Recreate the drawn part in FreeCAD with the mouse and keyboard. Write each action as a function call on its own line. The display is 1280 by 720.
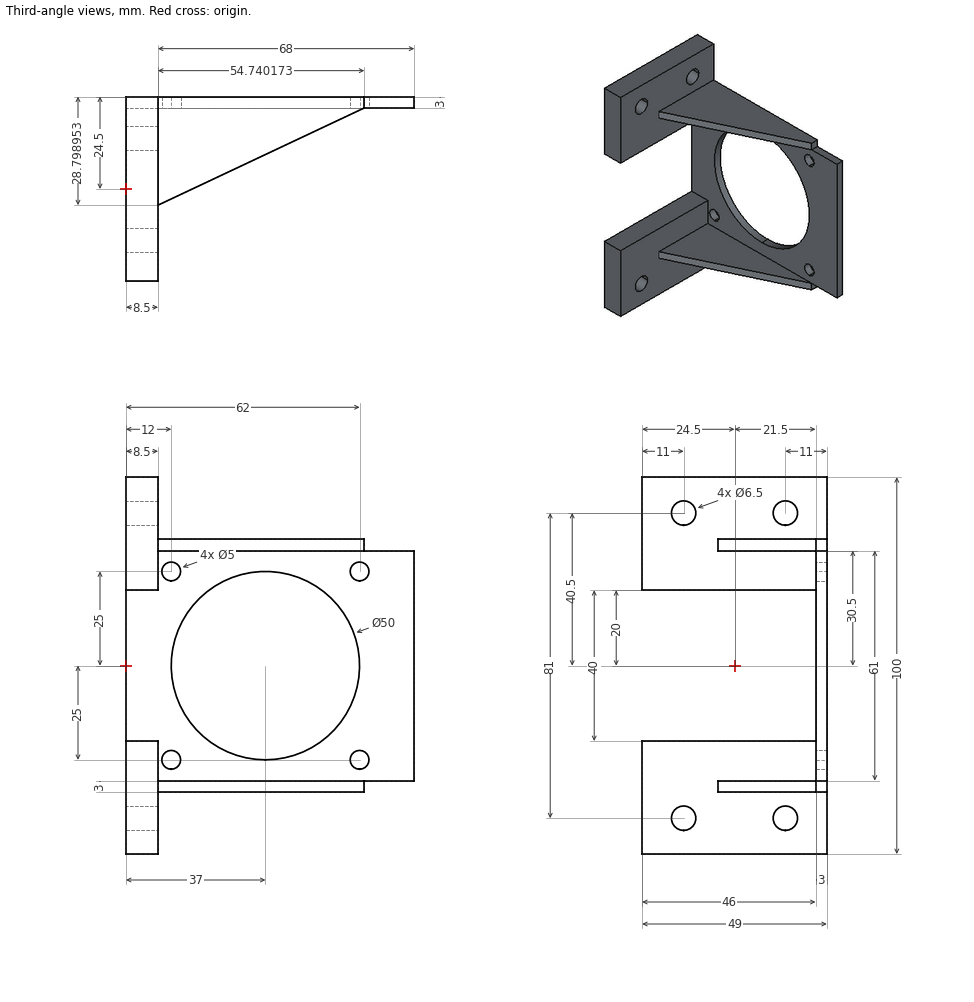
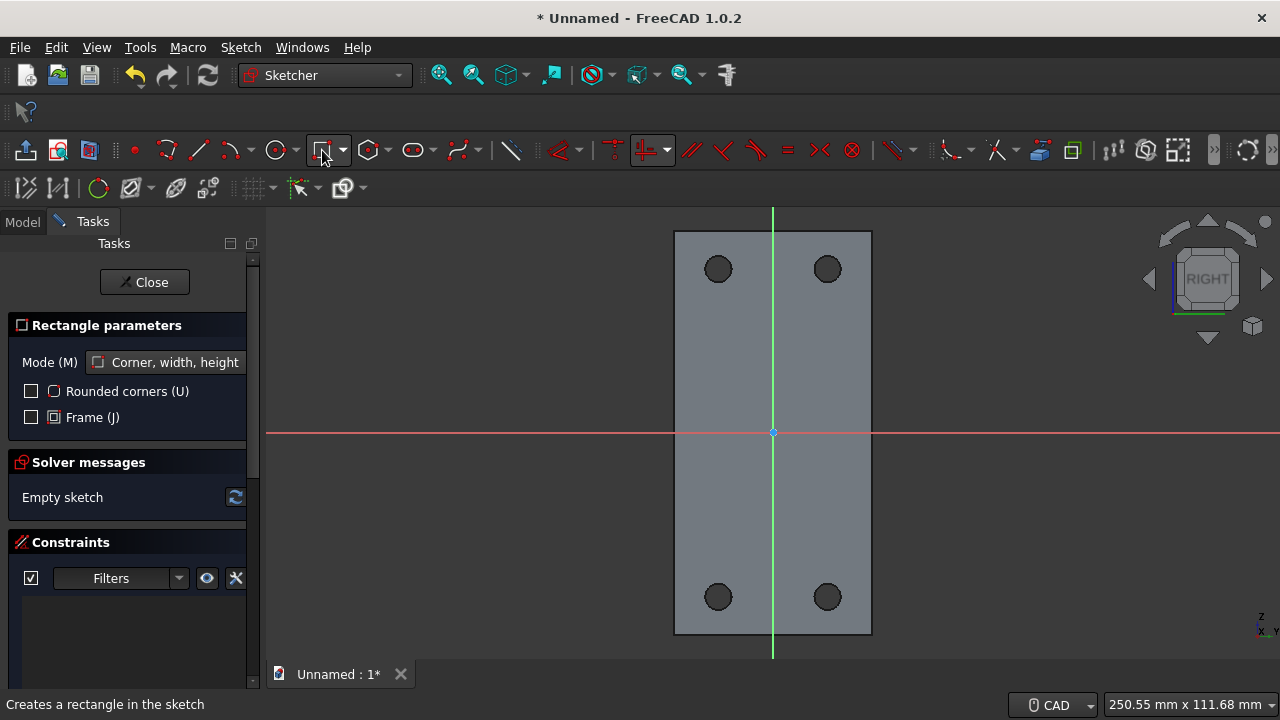
scroll(860, 310, up, 2)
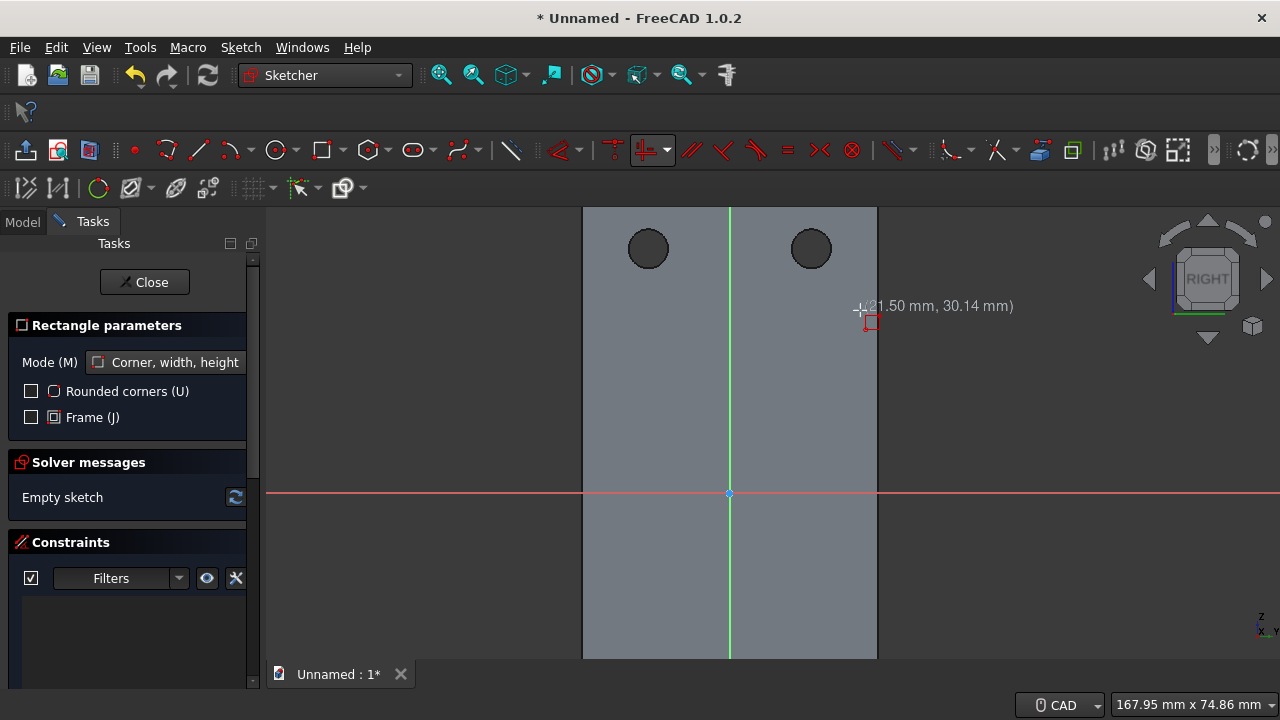
click(860, 309)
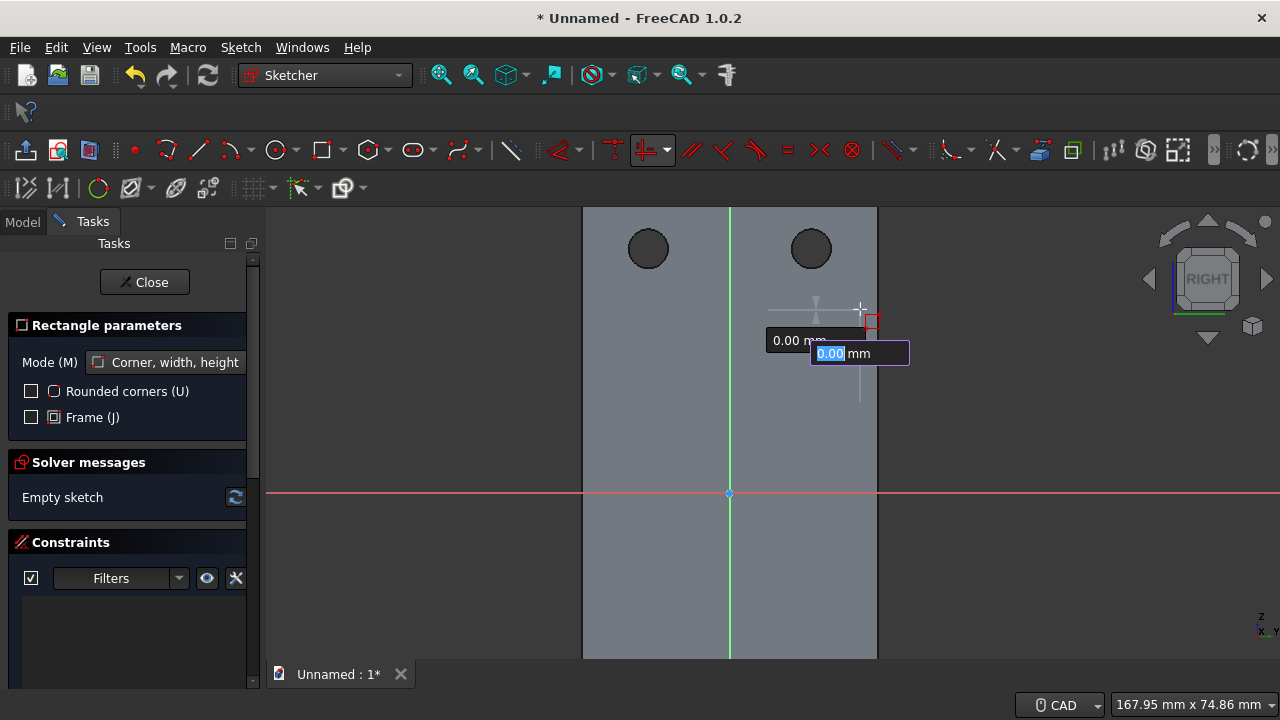
scroll(294, 235, down, 1)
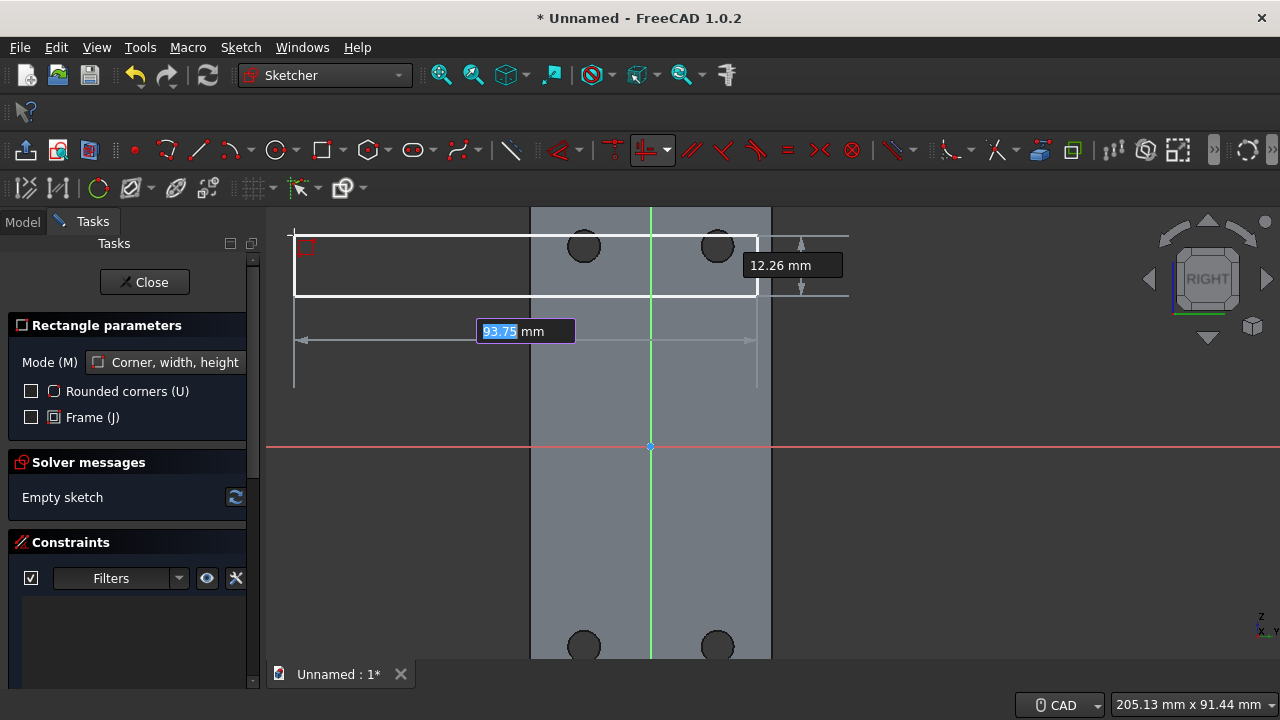
click(772, 597)
key(Escape)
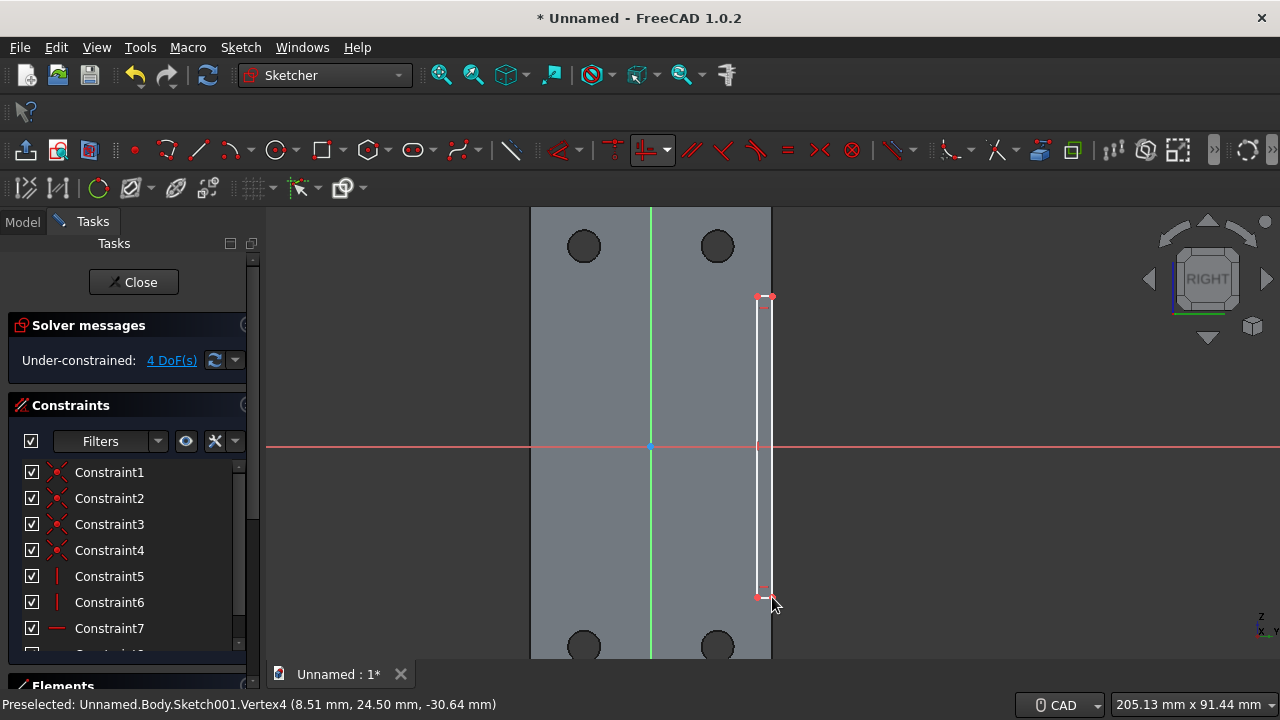
click(558, 150)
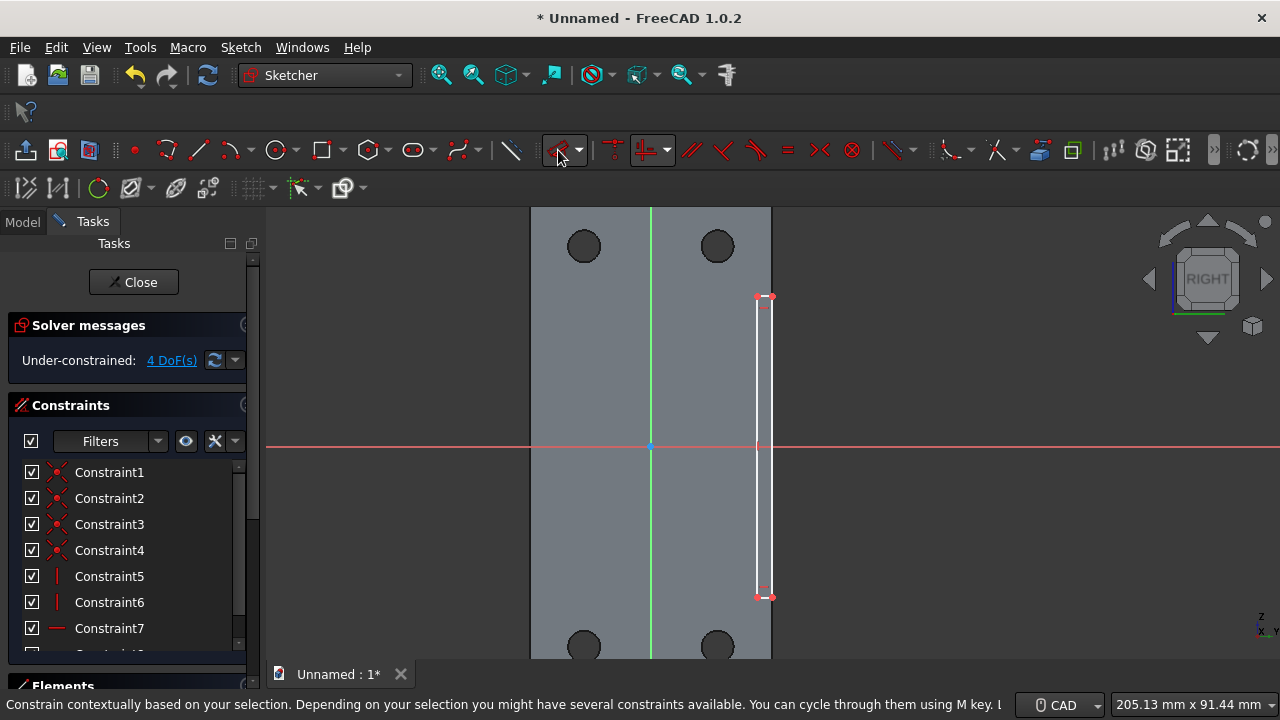
scroll(765, 598, up, 5)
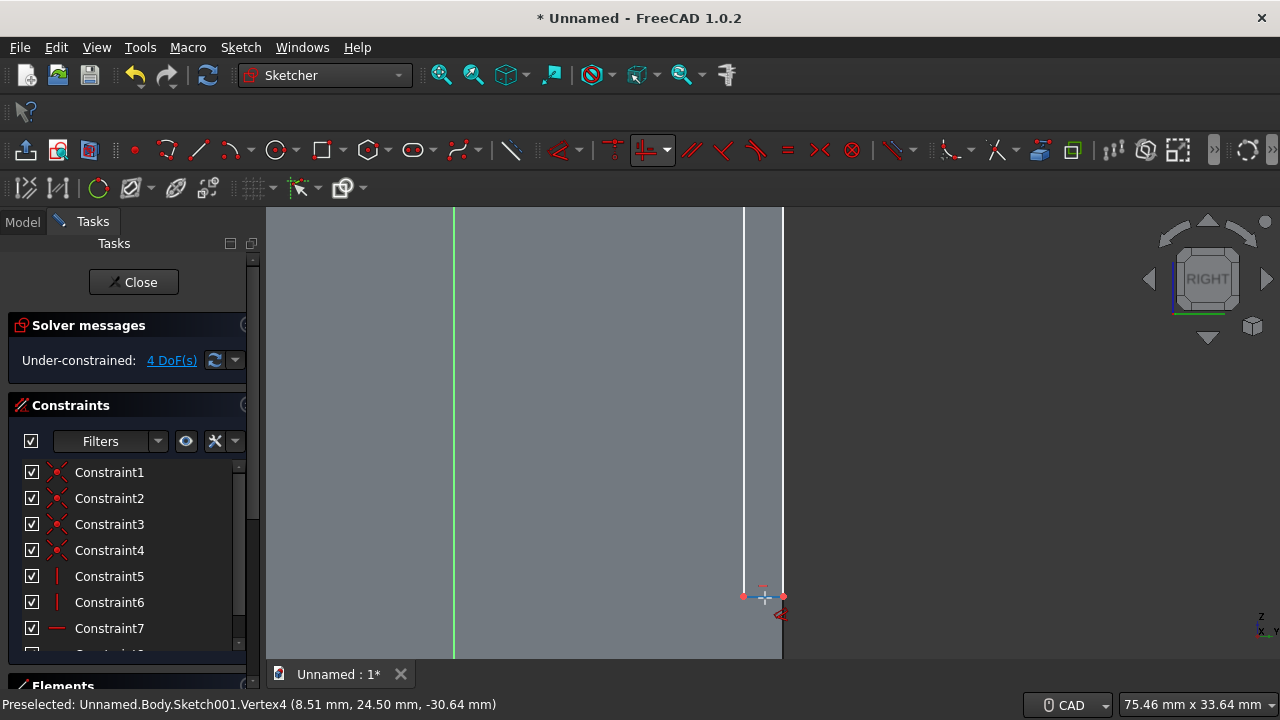
click(763, 597)
click(763, 631)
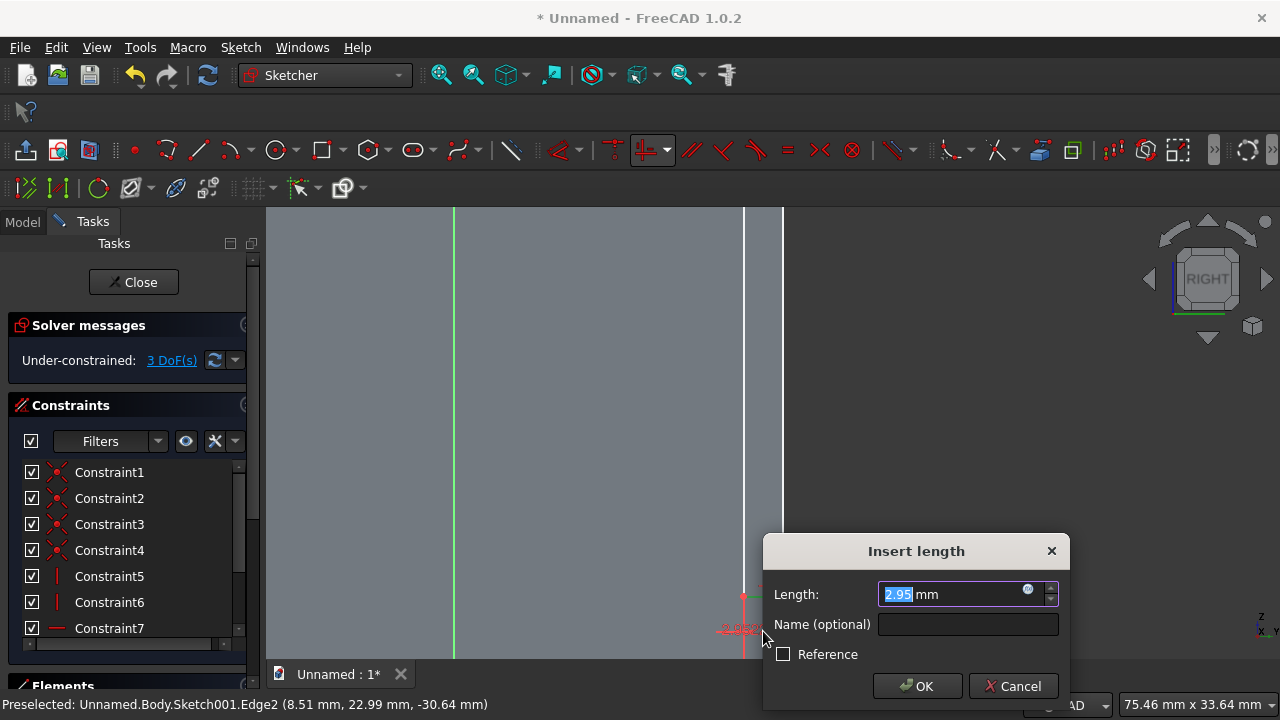
text(3)
key(Return)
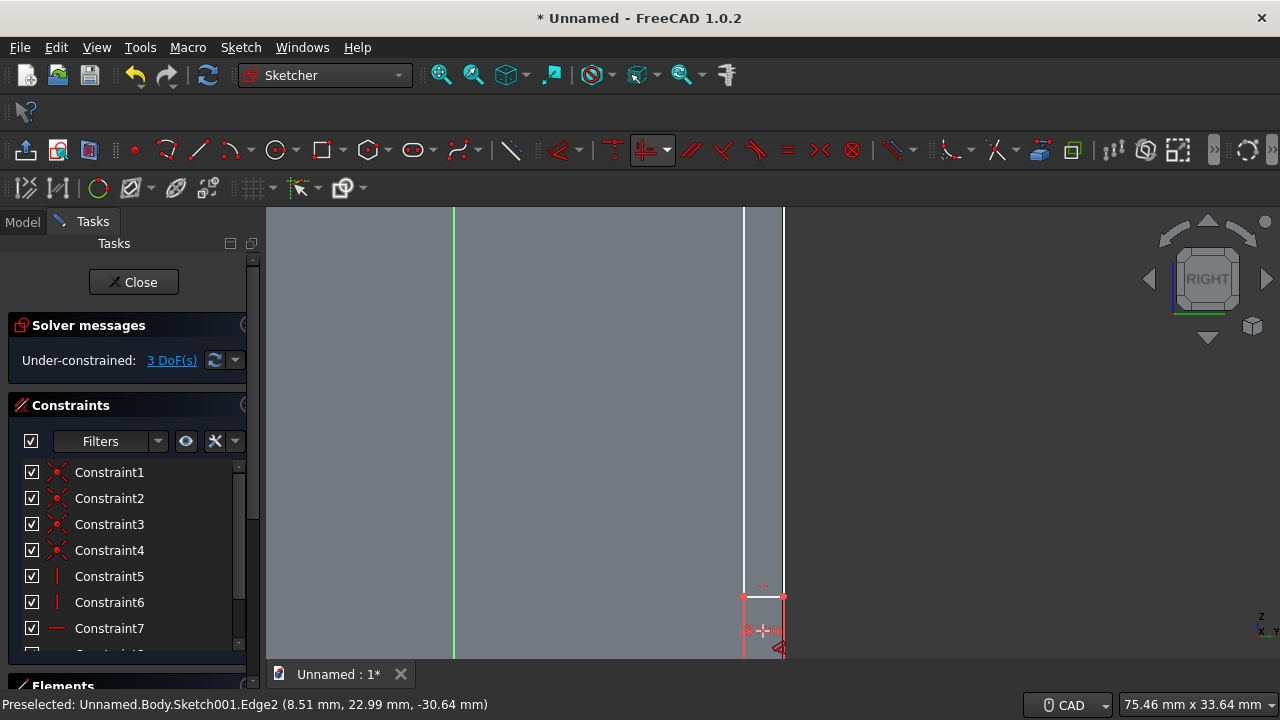
click(744, 351)
click(710, 416)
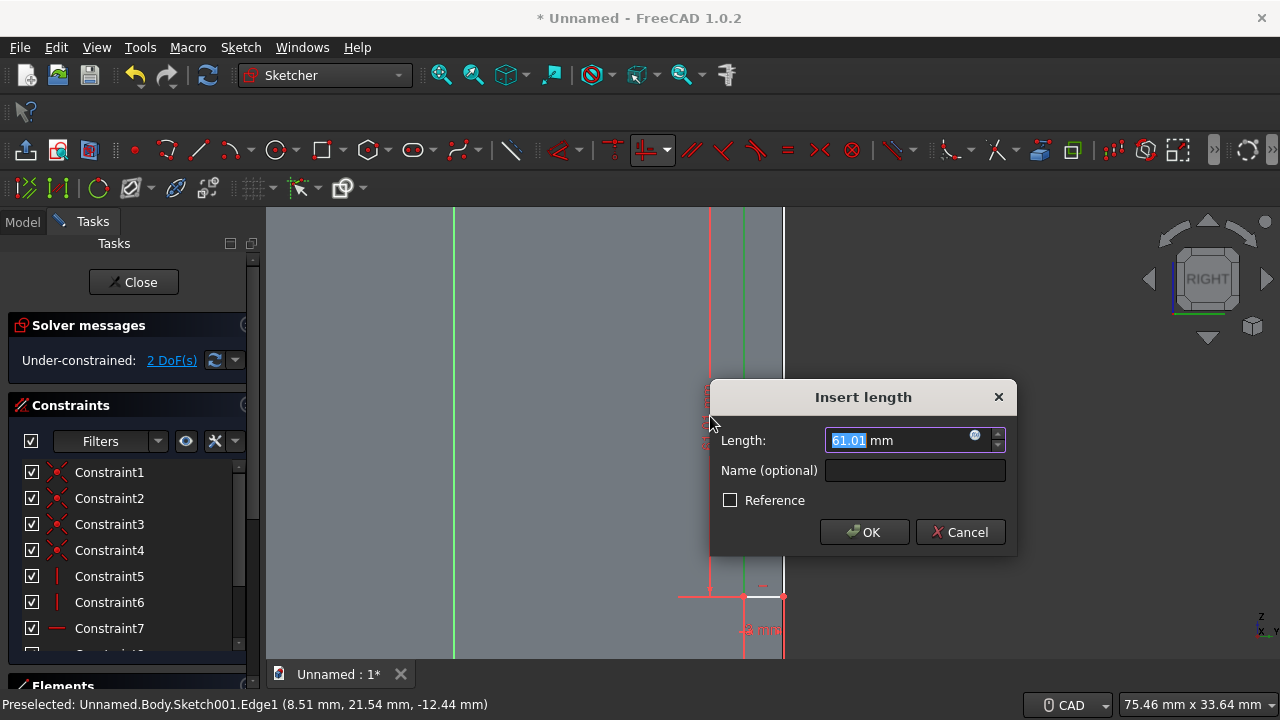
text(61)
key(Return)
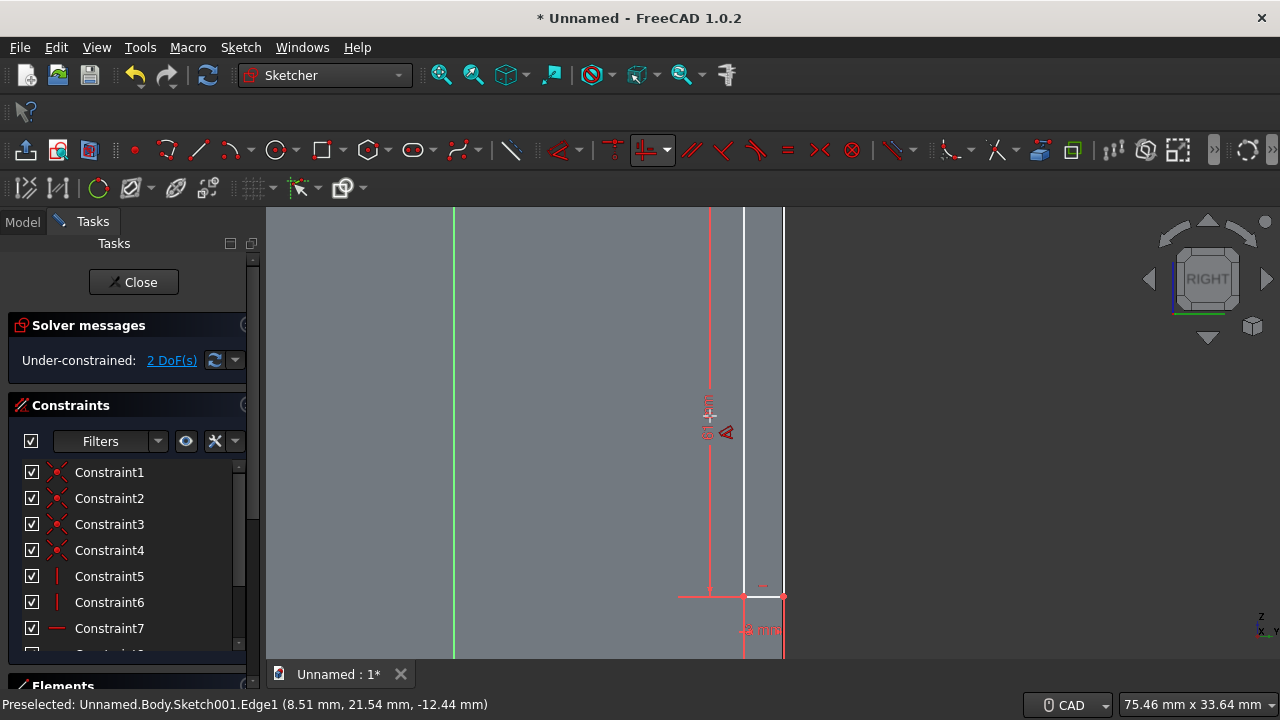
scroll(754, 577, down, 5)